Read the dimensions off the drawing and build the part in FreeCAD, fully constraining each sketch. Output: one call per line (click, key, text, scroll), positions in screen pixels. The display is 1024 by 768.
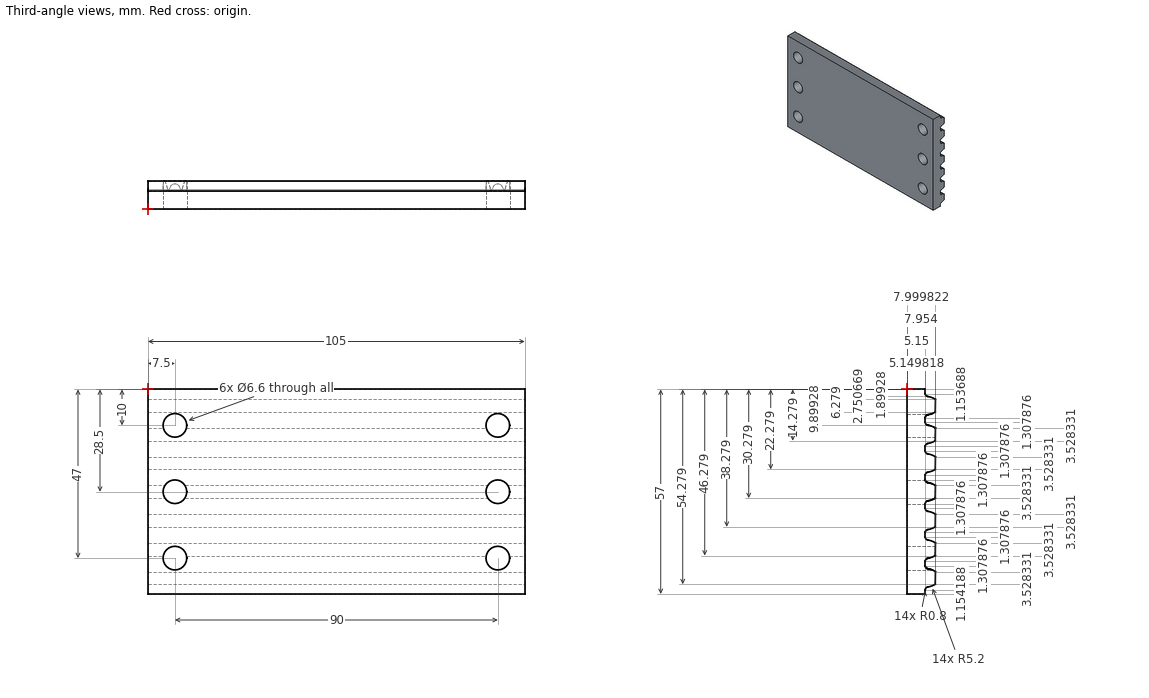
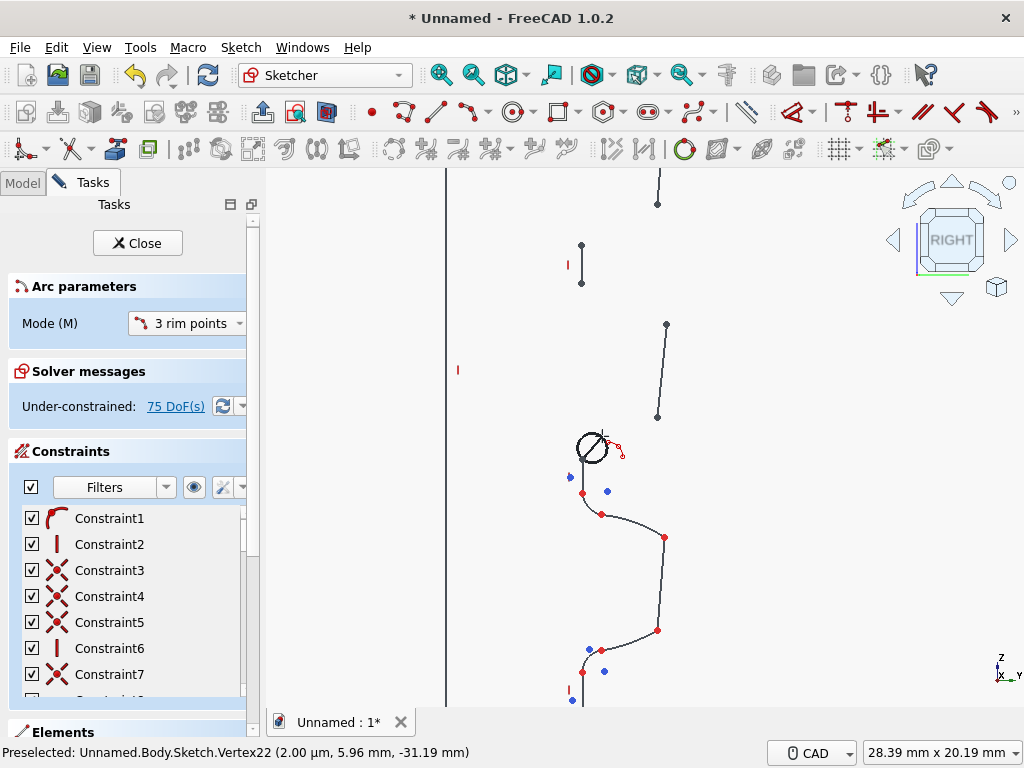
scroll(588, 443, up, 6)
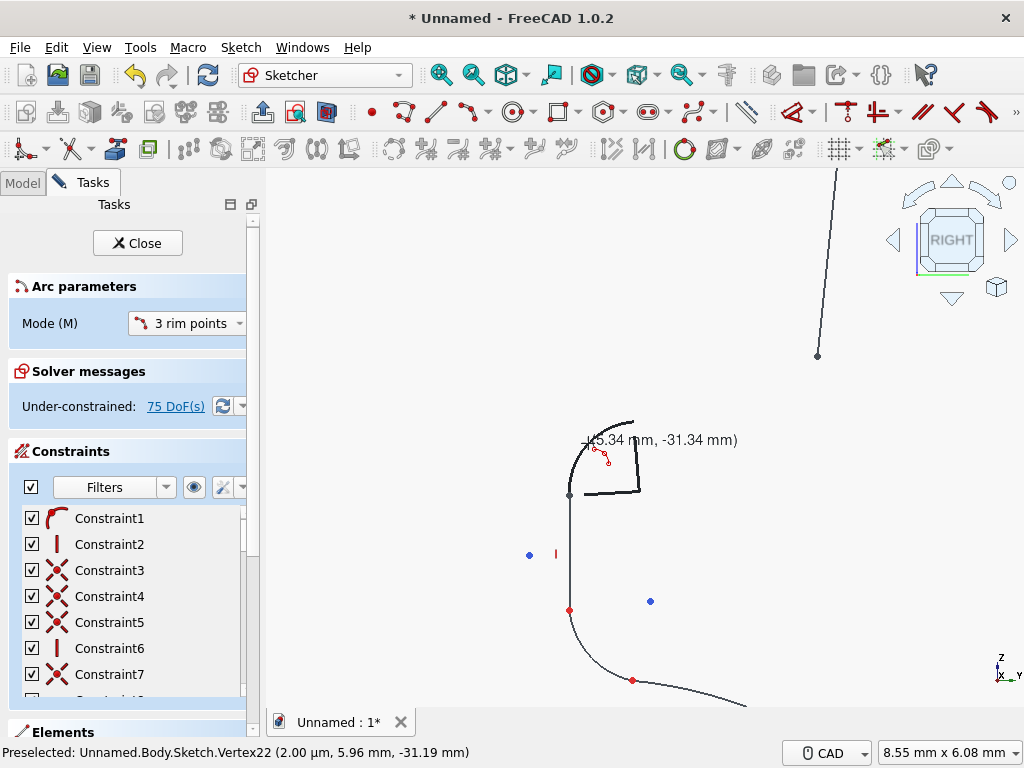
click(588, 443)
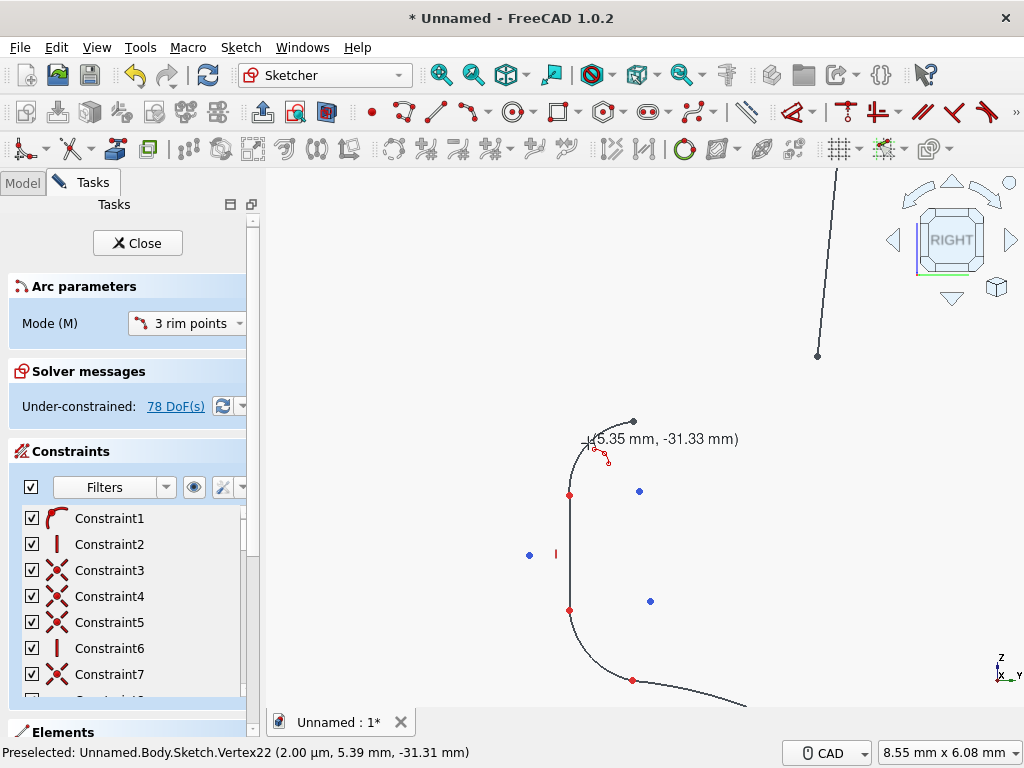
scroll(585, 457, down, 13)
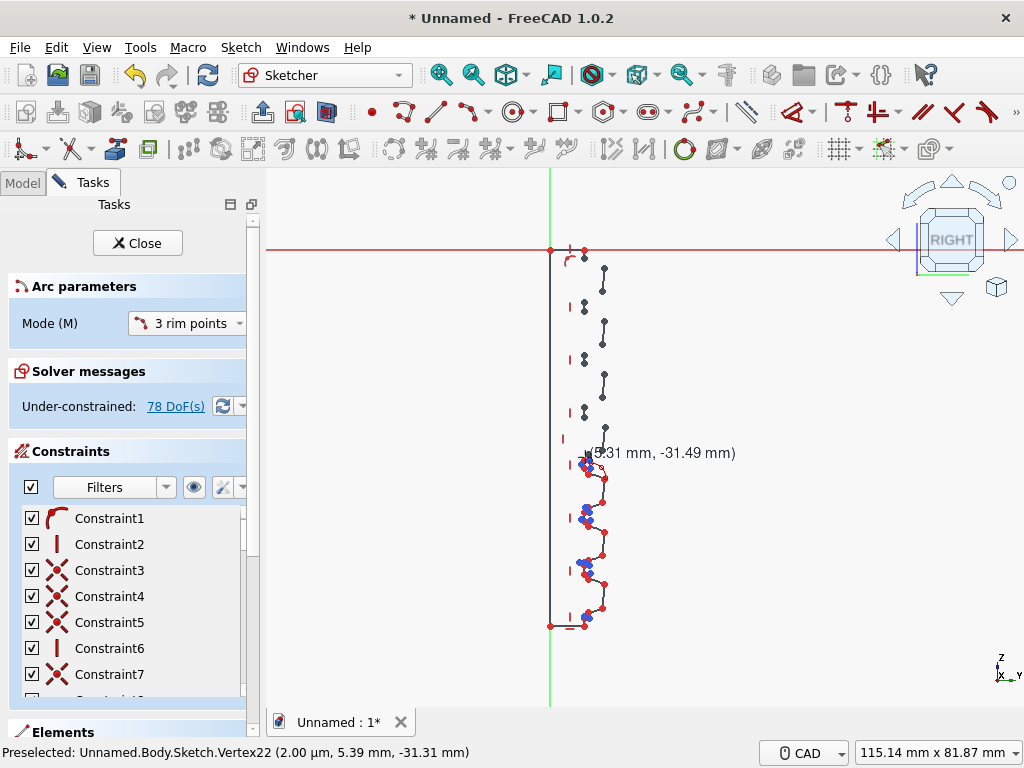
scroll(589, 455, up, 6)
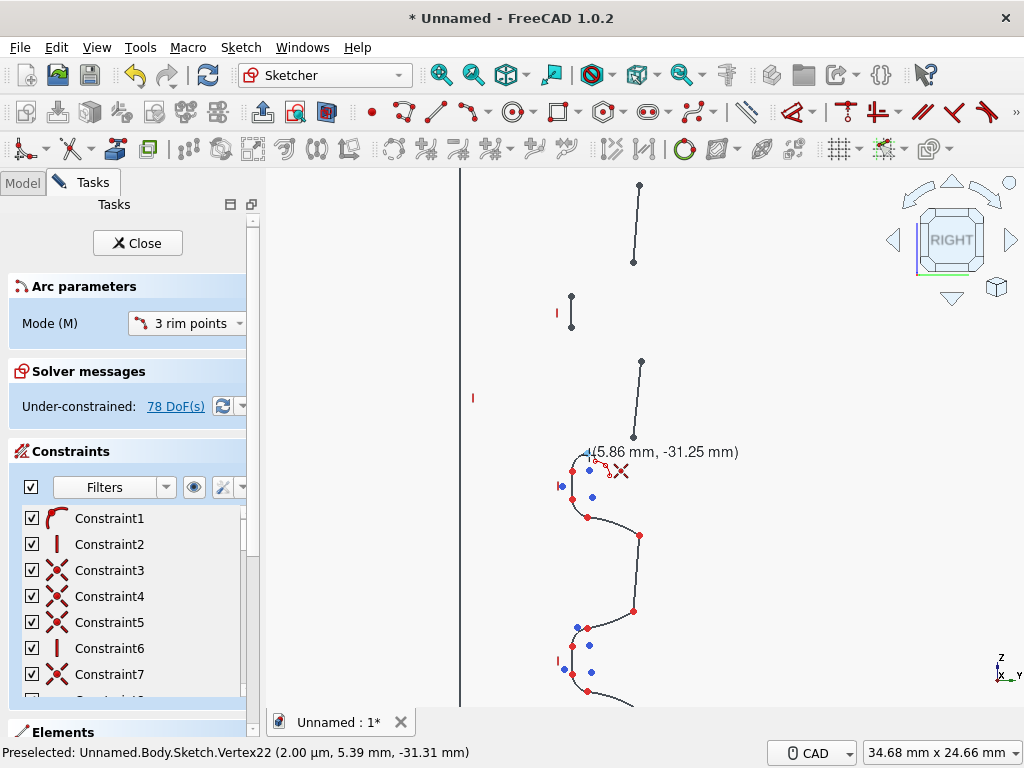
click(588, 453)
click(633, 437)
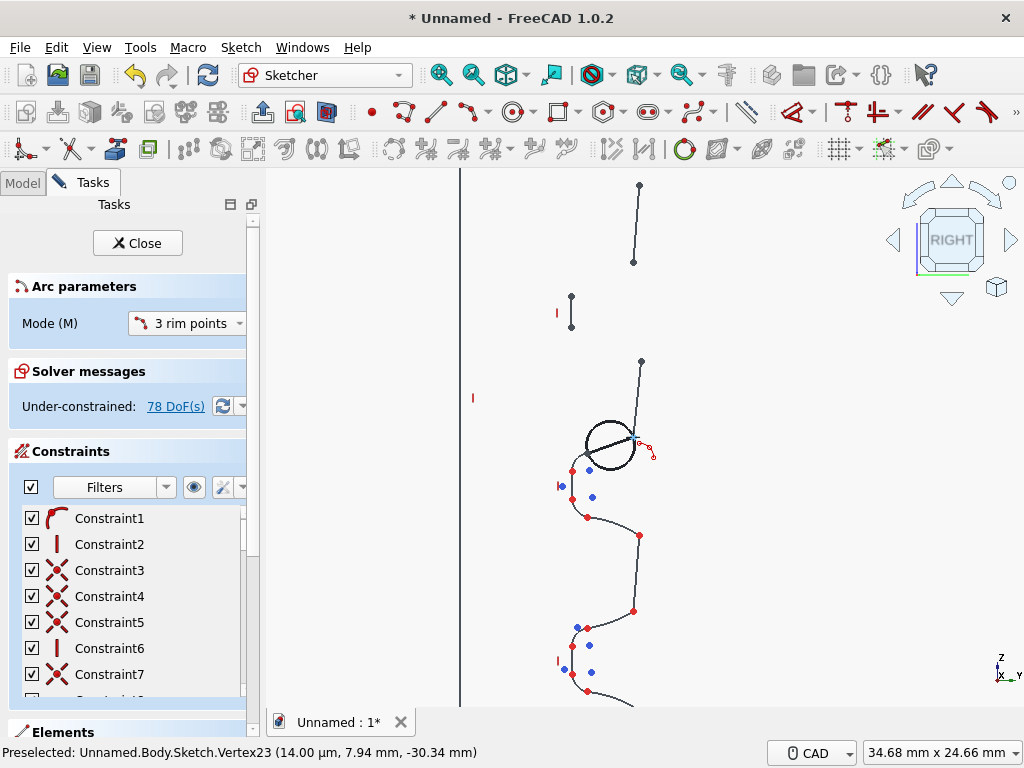
scroll(612, 447, up, 9)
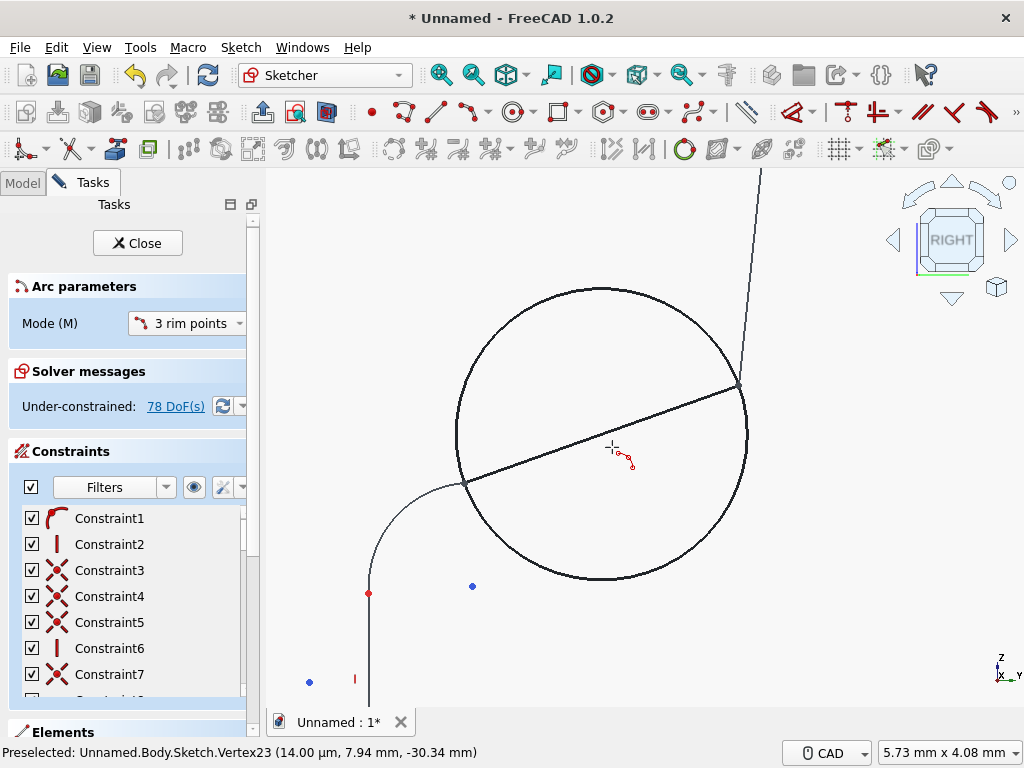
click(607, 444)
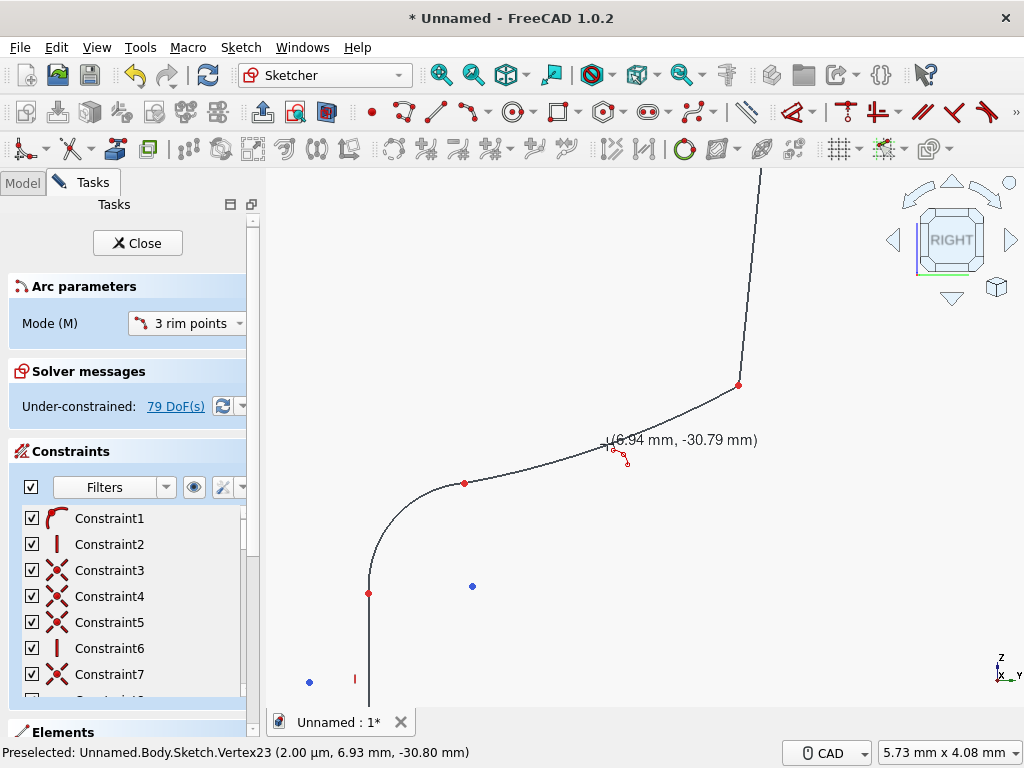
scroll(595, 453, down, 15)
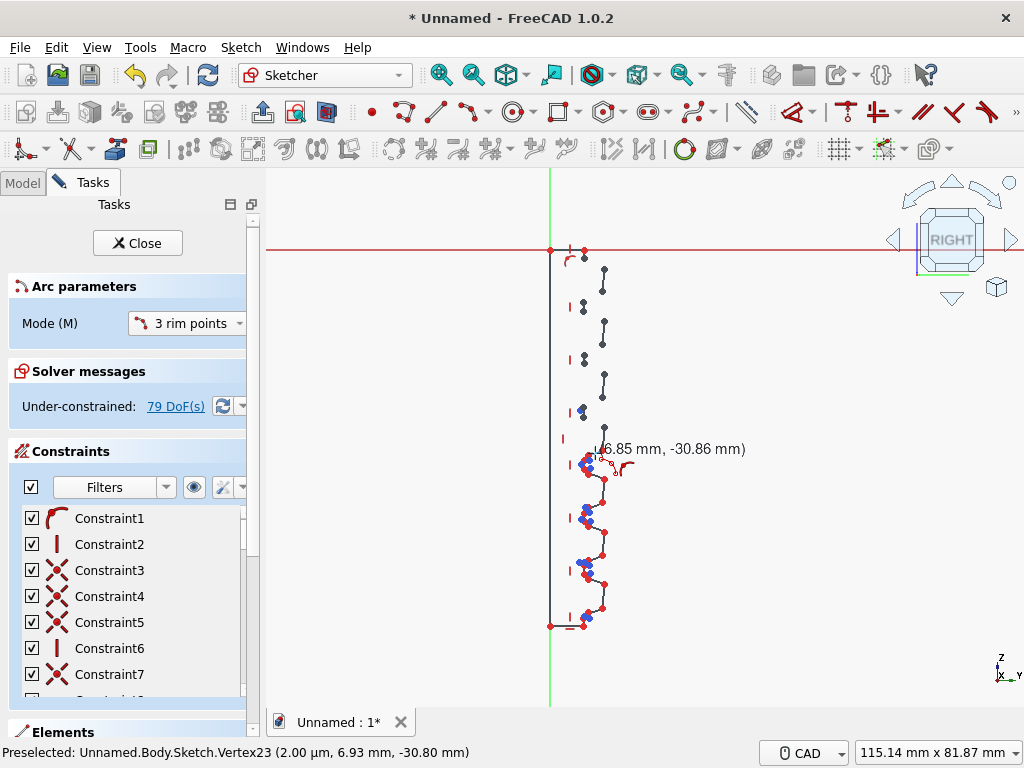
scroll(603, 427, up, 2)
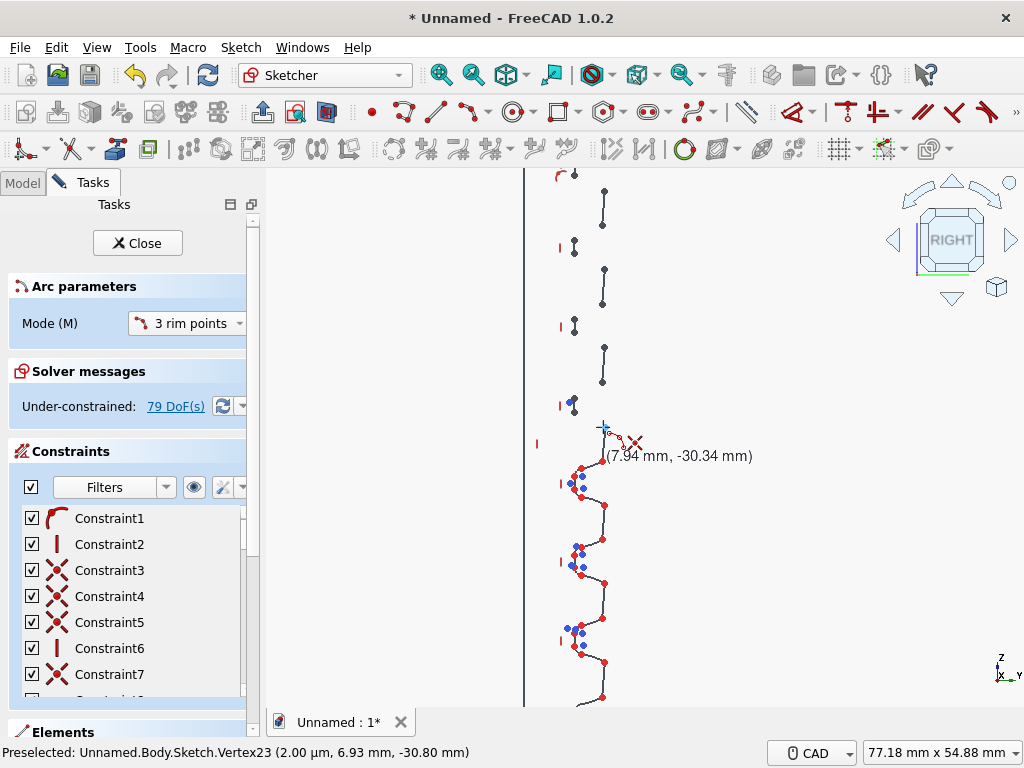
click(606, 427)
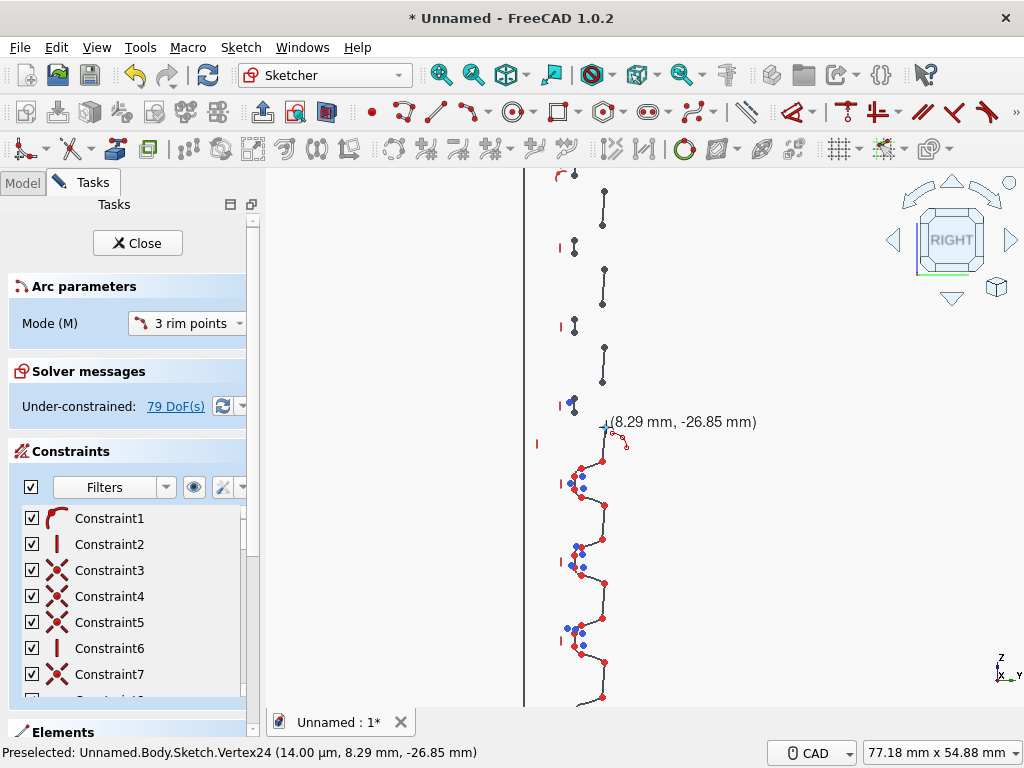
scroll(582, 418, up, 5)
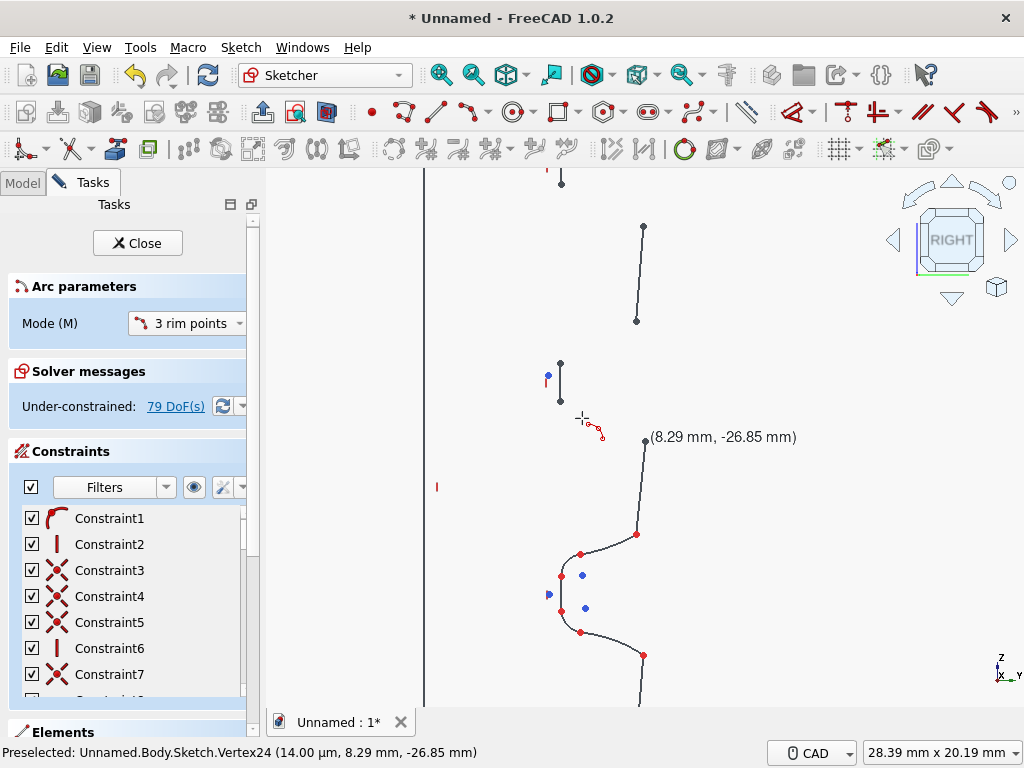
click(580, 418)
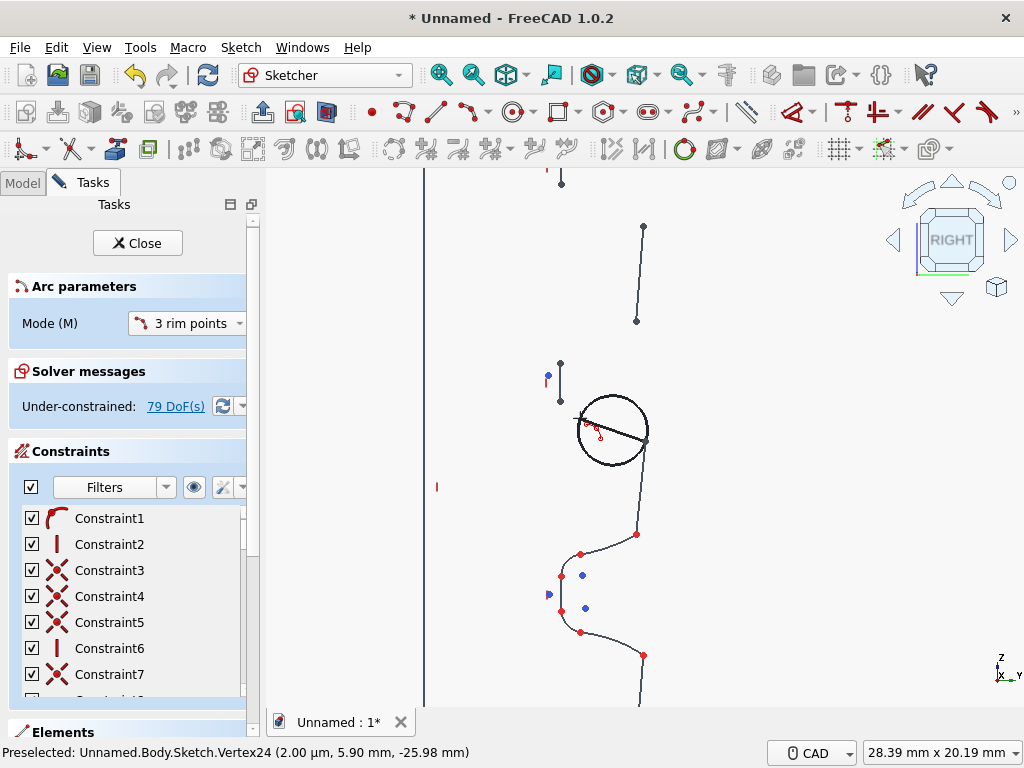
scroll(610, 425, up, 8)